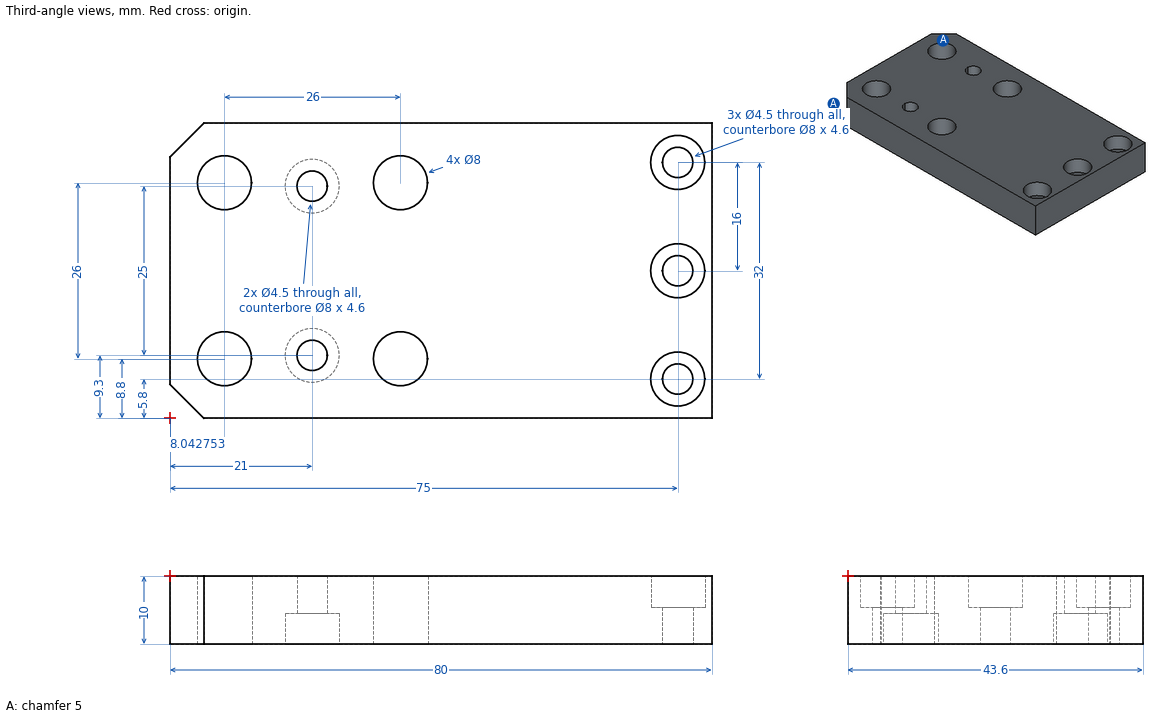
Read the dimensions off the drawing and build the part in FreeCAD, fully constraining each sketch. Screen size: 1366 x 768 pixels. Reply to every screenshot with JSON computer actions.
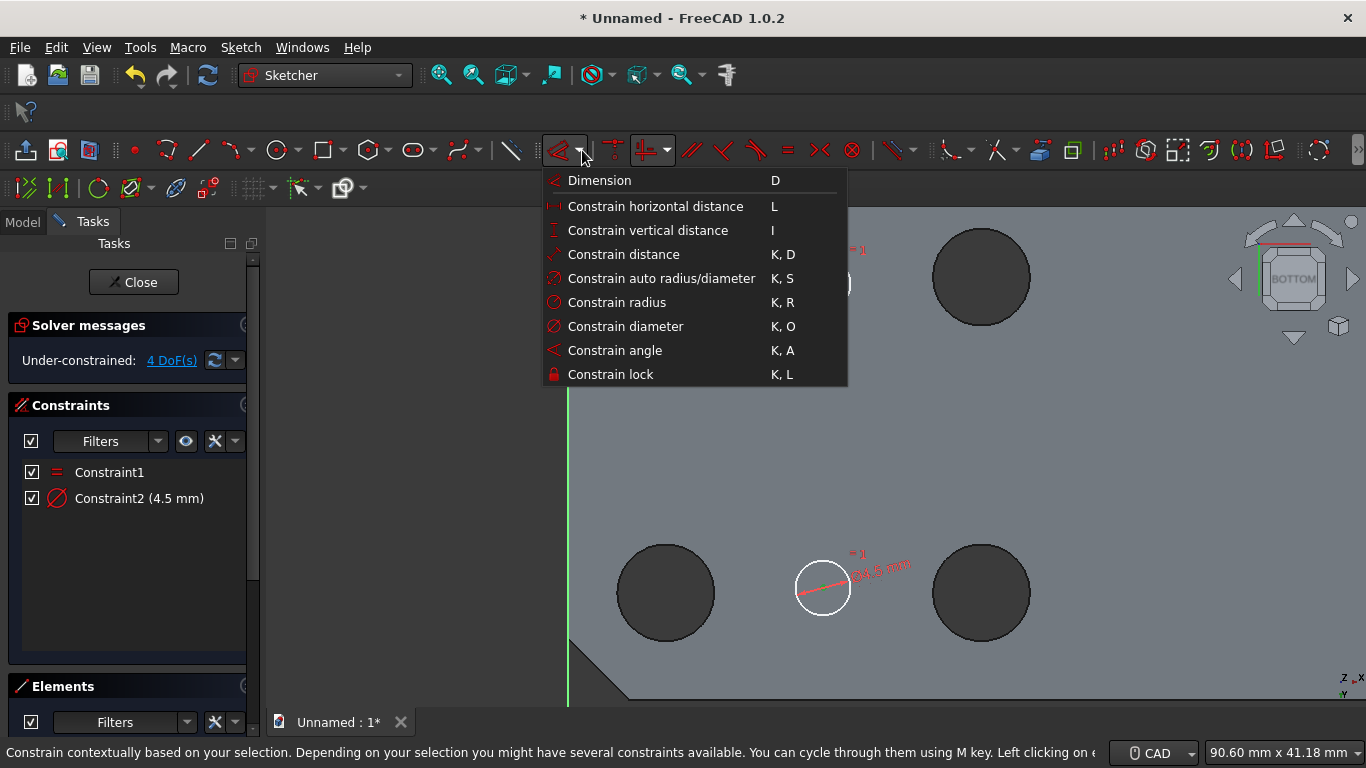
{"action": "left_click", "coordinate": [695, 206]}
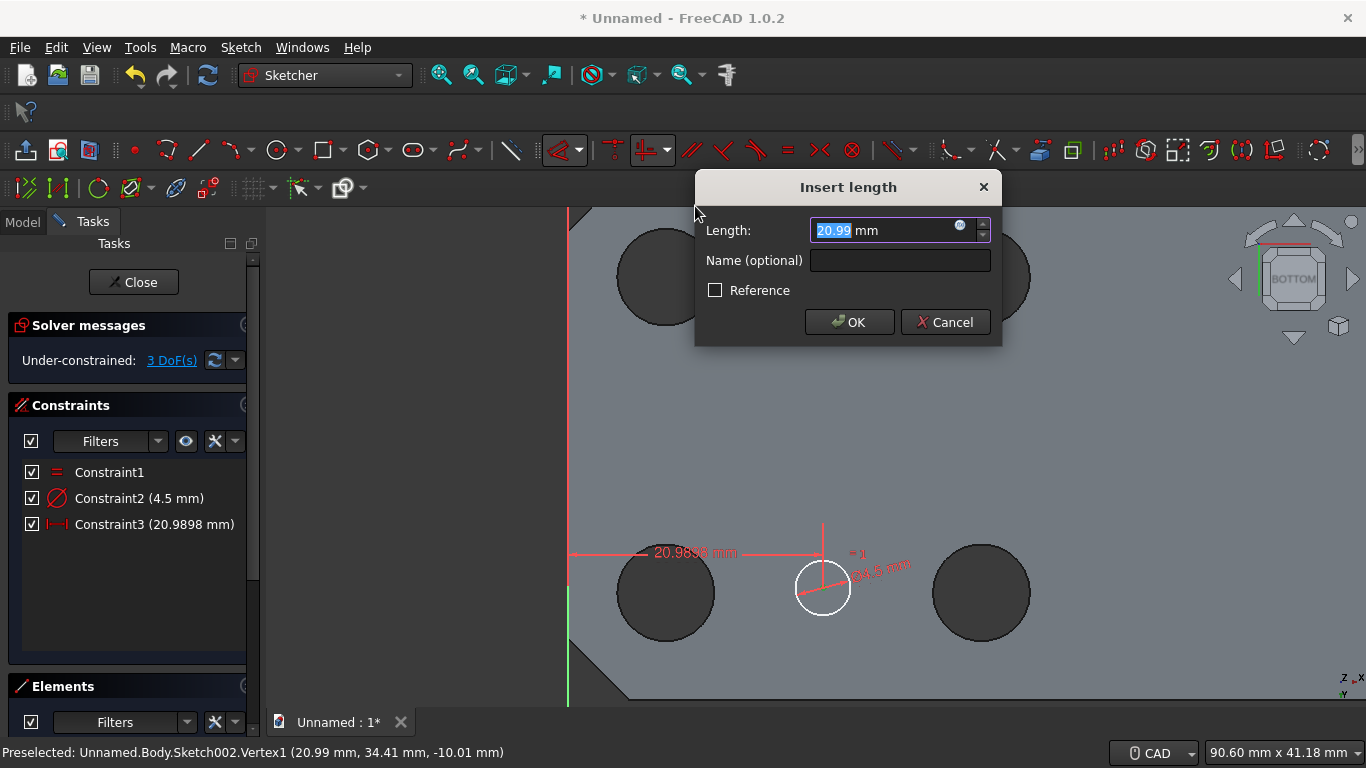
{"action": "type", "text": "21"}
{"action": "key", "text": "Return"}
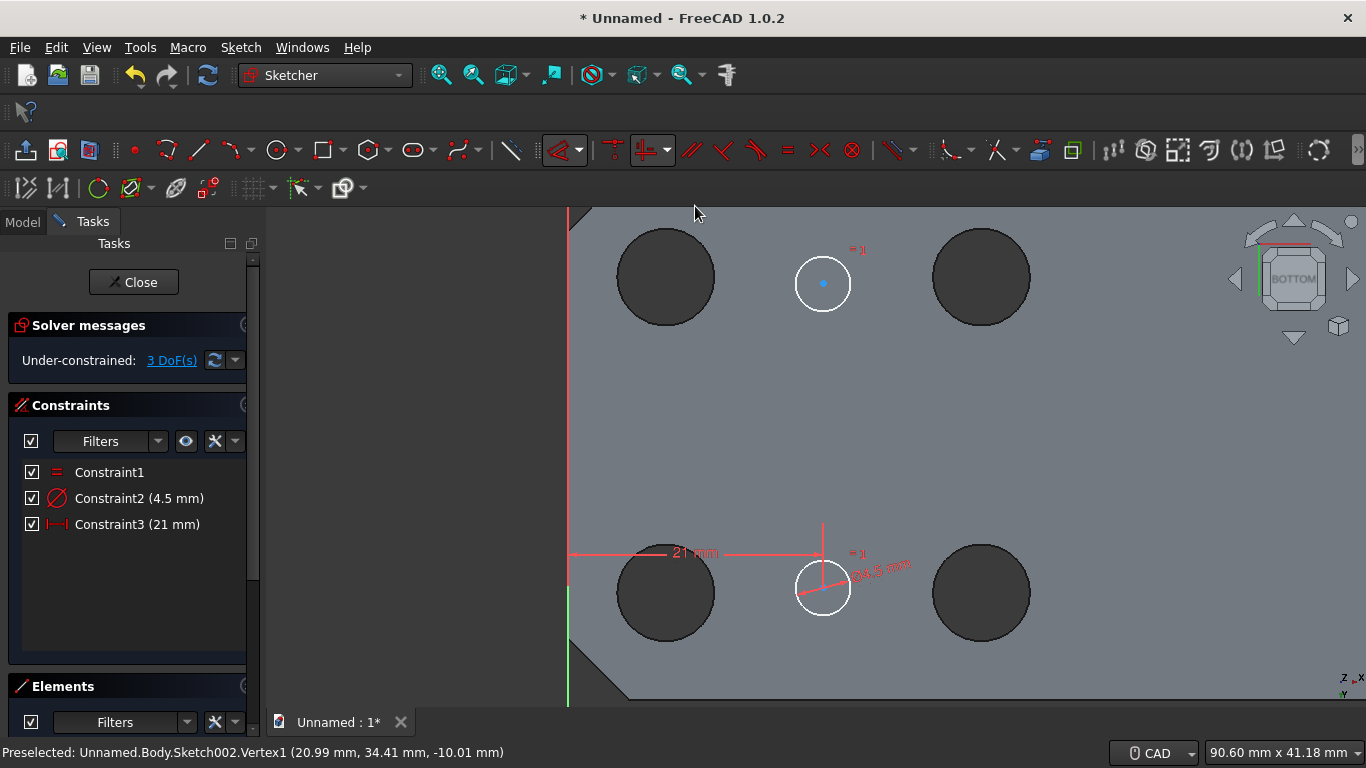
{"action": "left_click", "coordinate": [823, 284]}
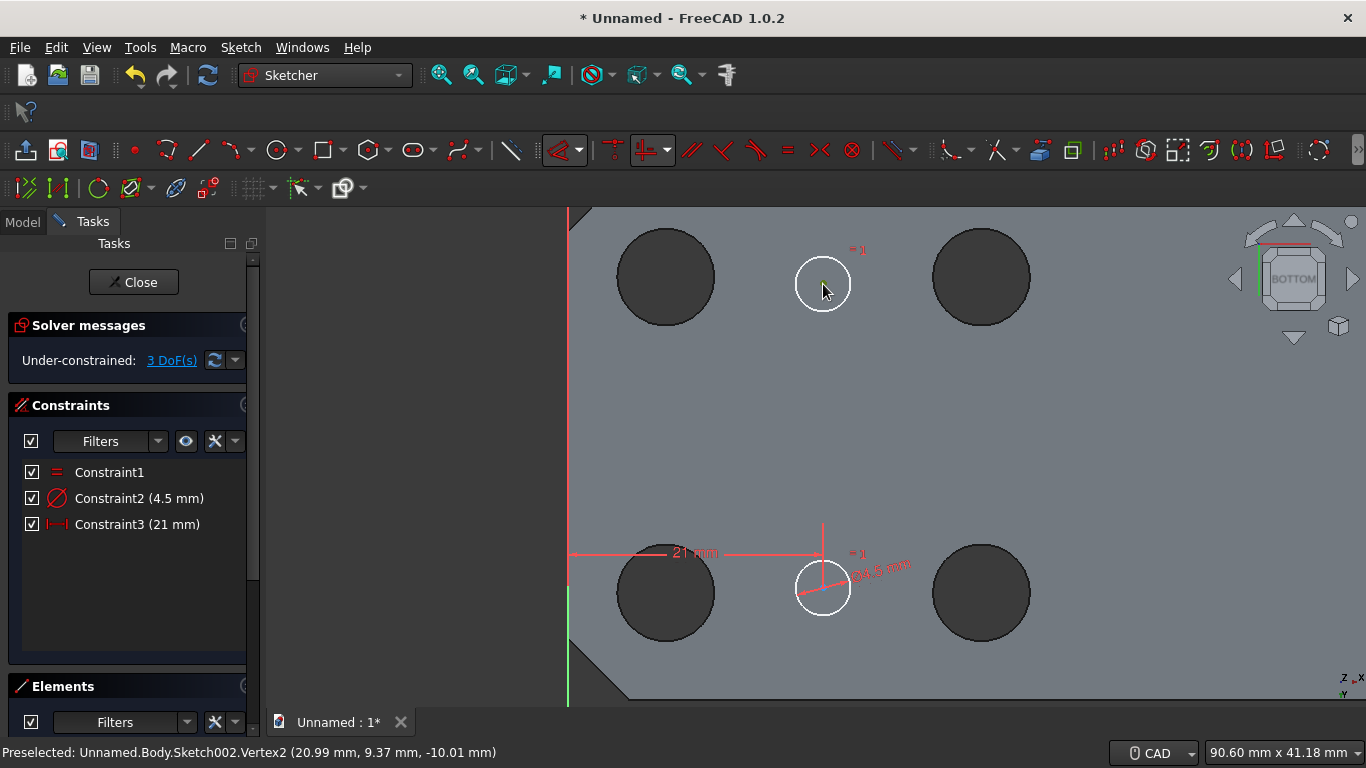
{"action": "key", "text": "l"}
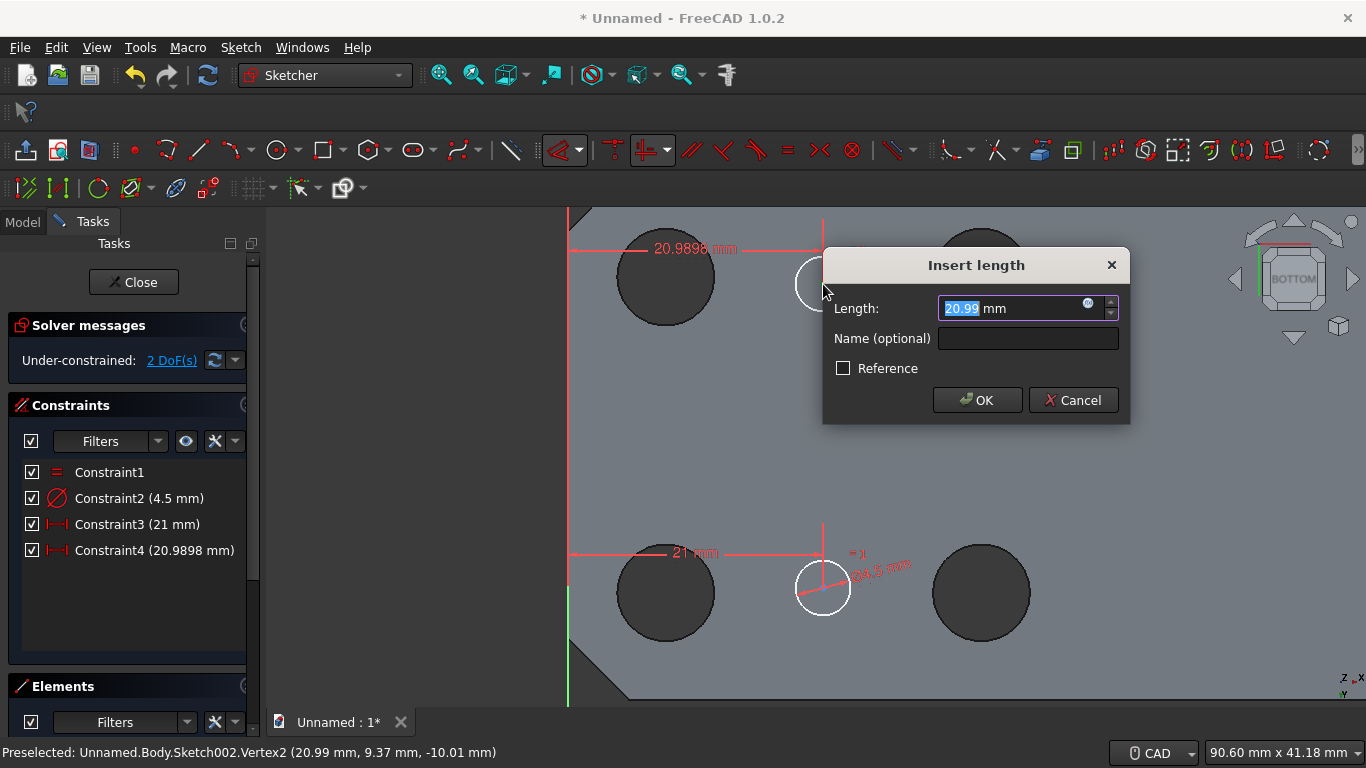
{"action": "type", "text": "21"}
{"action": "key", "text": "Return"}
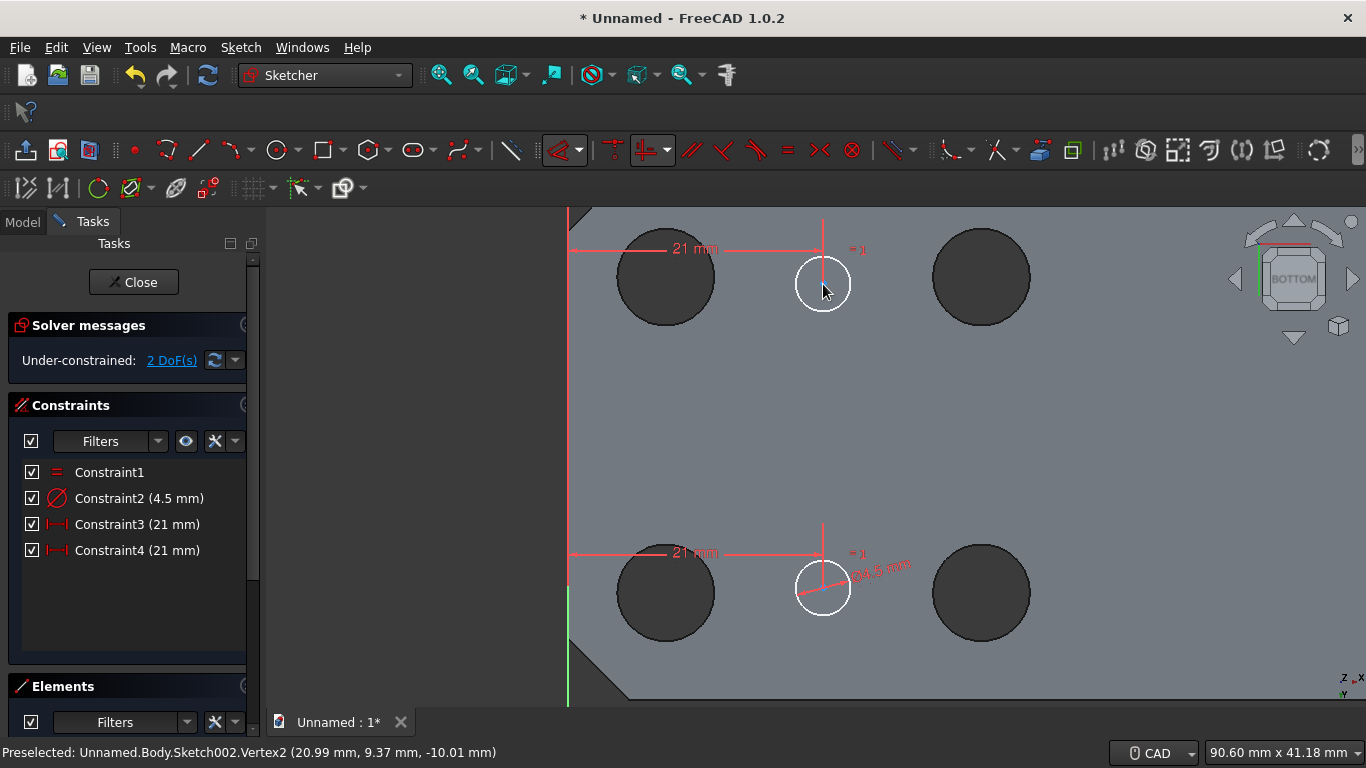
{"action": "left_click", "coordinate": [823, 284]}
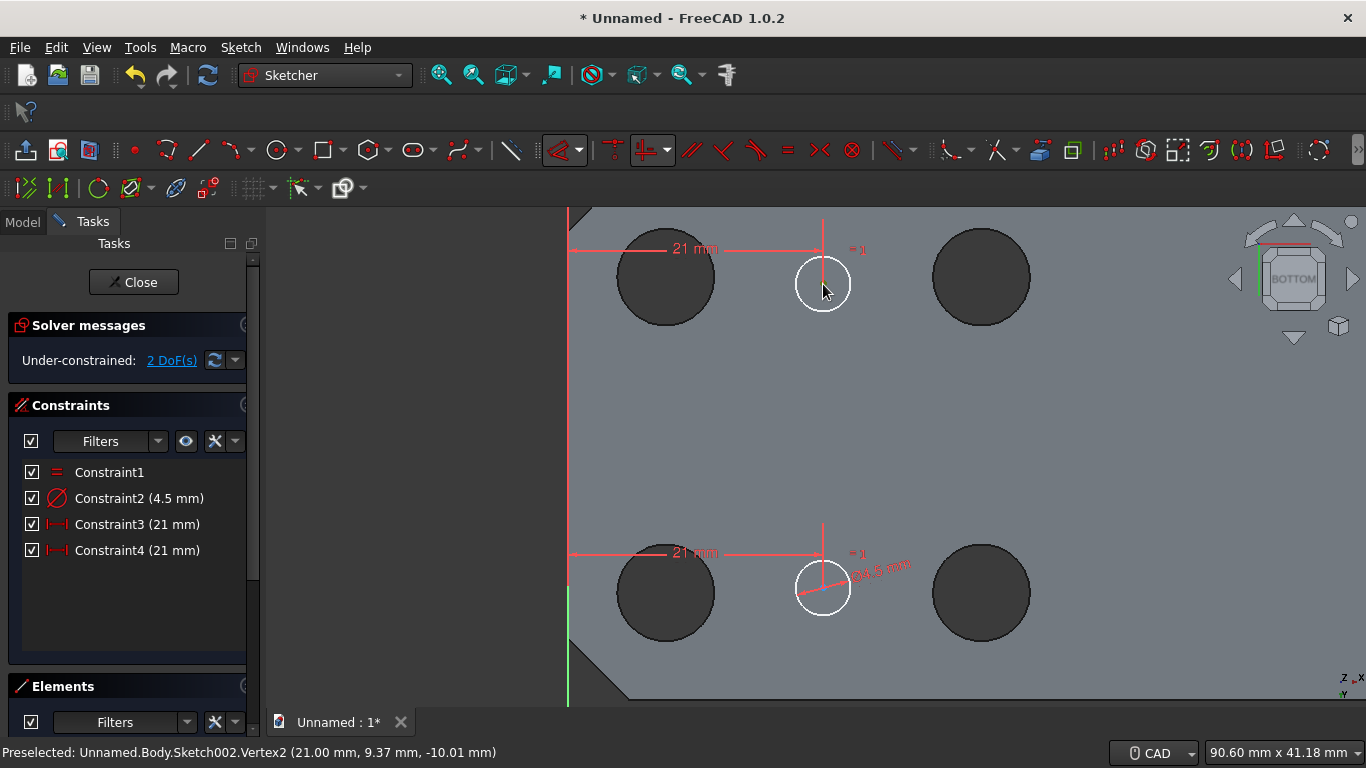
{"action": "key", "text": "i"}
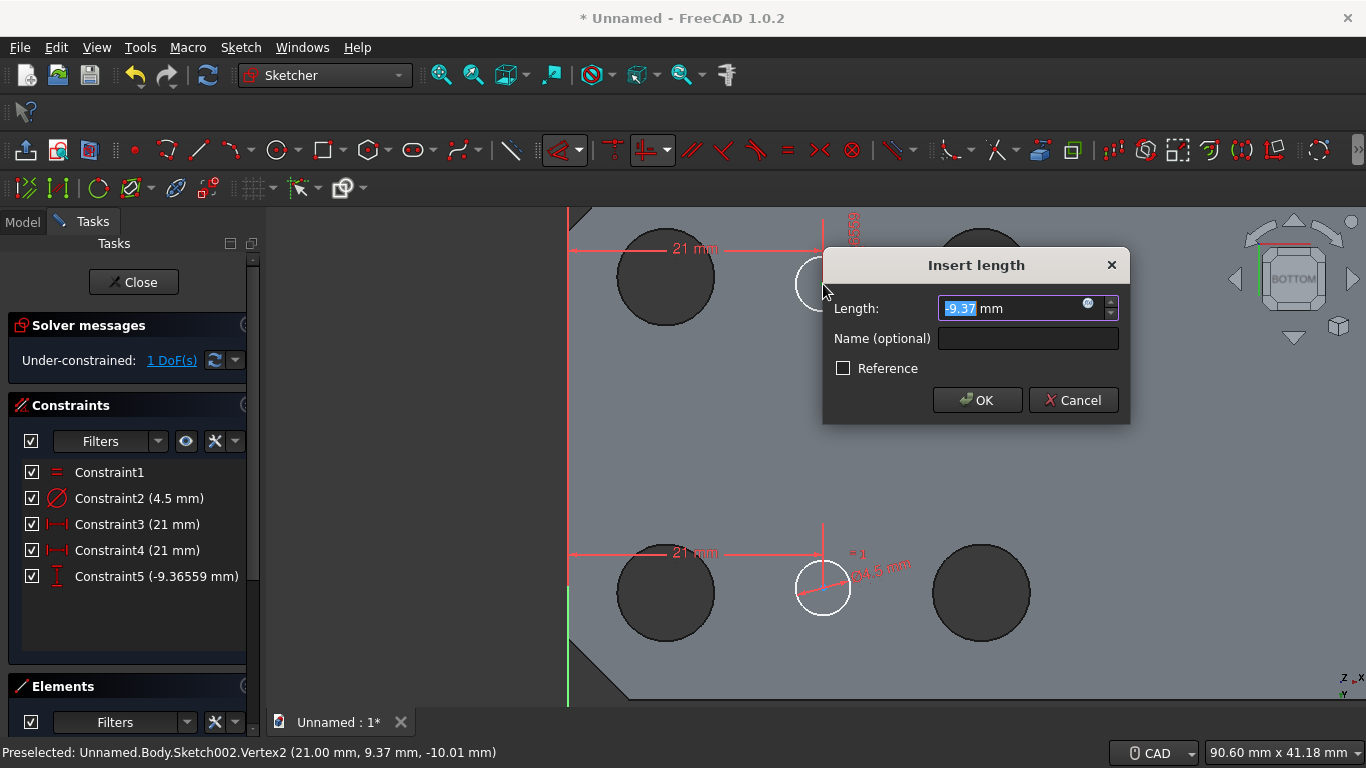
{"action": "type", "text": "-9.3"}
{"action": "key", "text": "Return"}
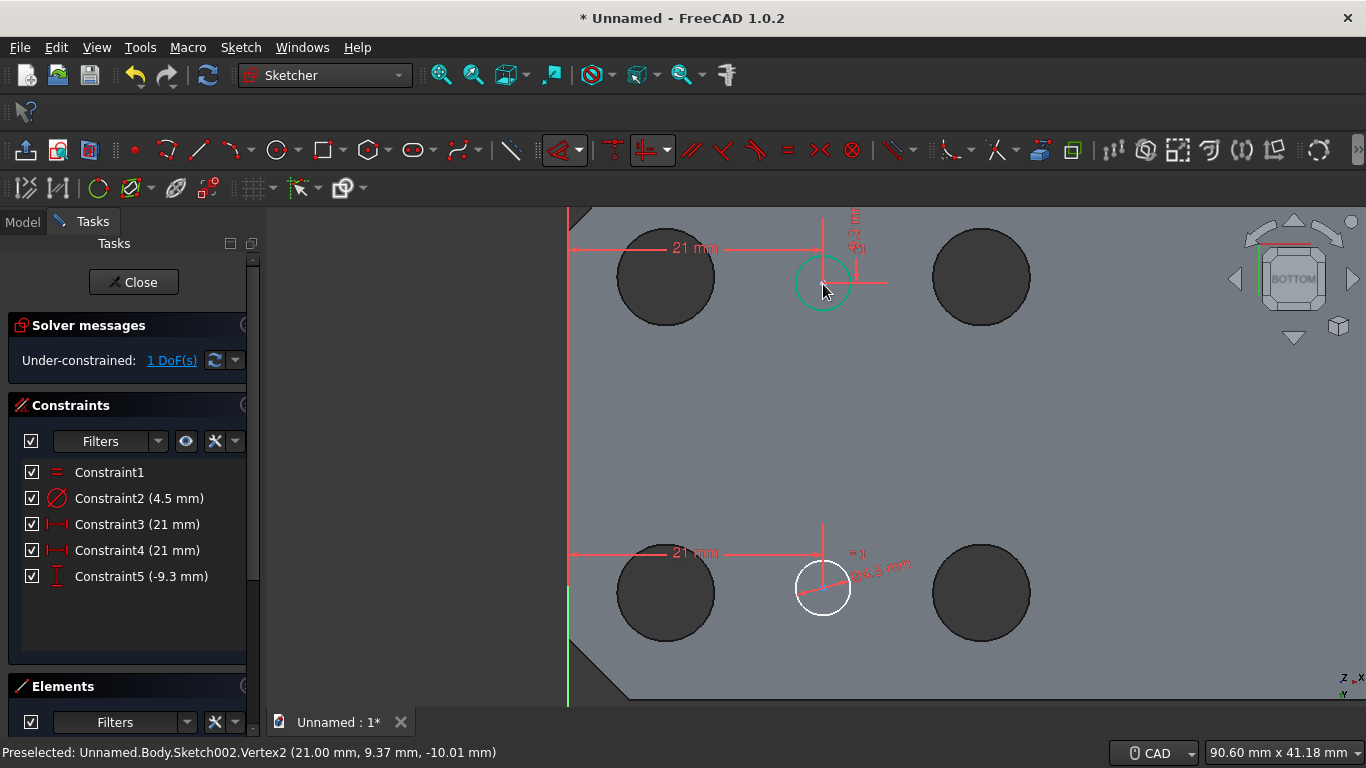
{"action": "left_click", "coordinate": [823, 588]}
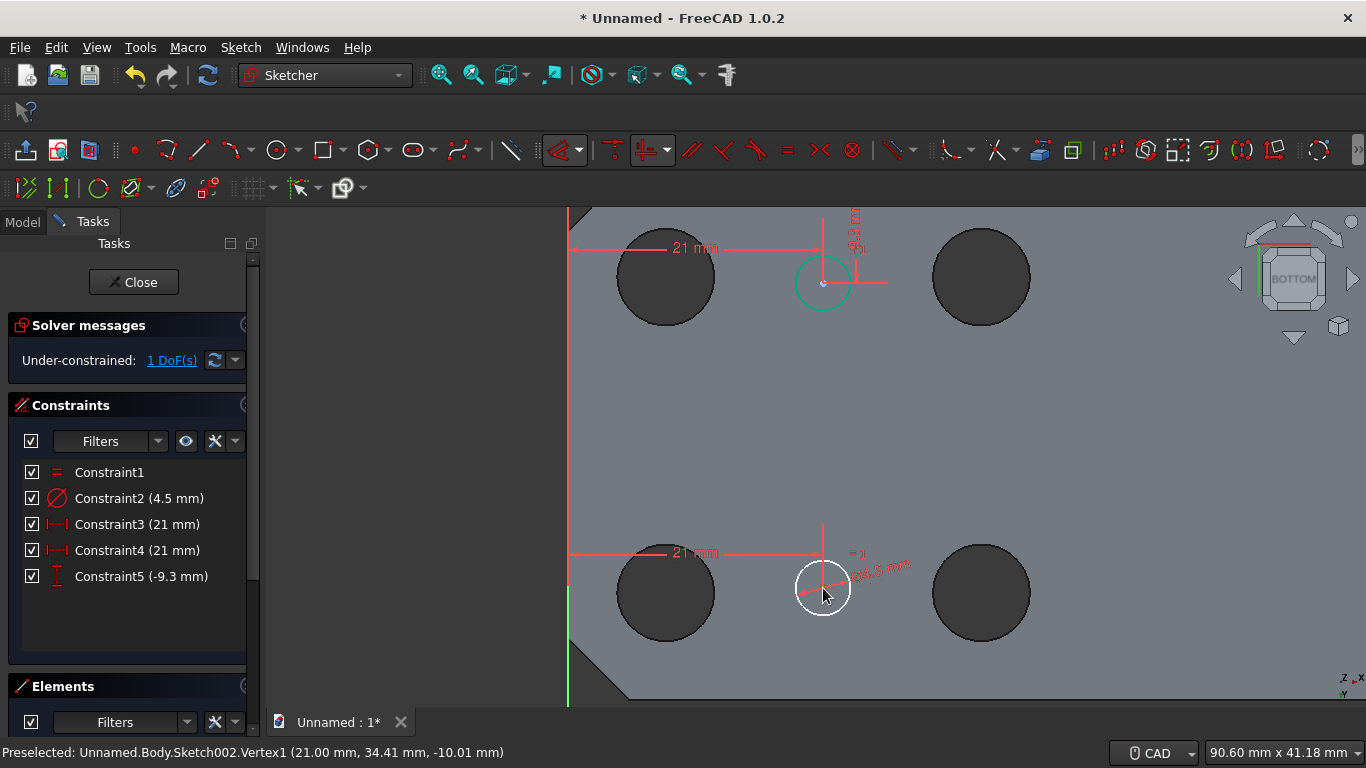
{"action": "left_click", "coordinate": [823, 283]}